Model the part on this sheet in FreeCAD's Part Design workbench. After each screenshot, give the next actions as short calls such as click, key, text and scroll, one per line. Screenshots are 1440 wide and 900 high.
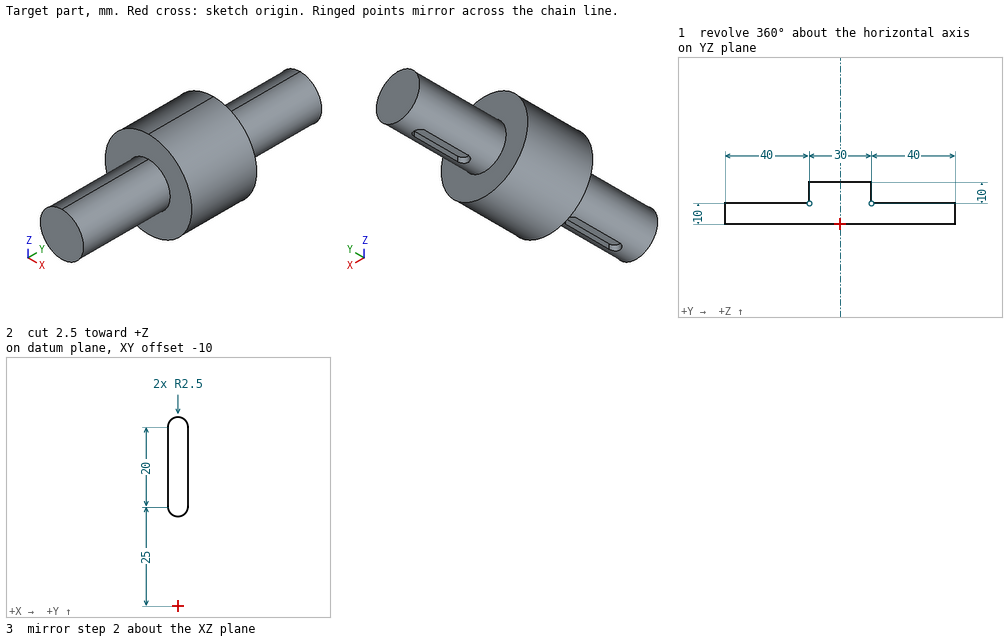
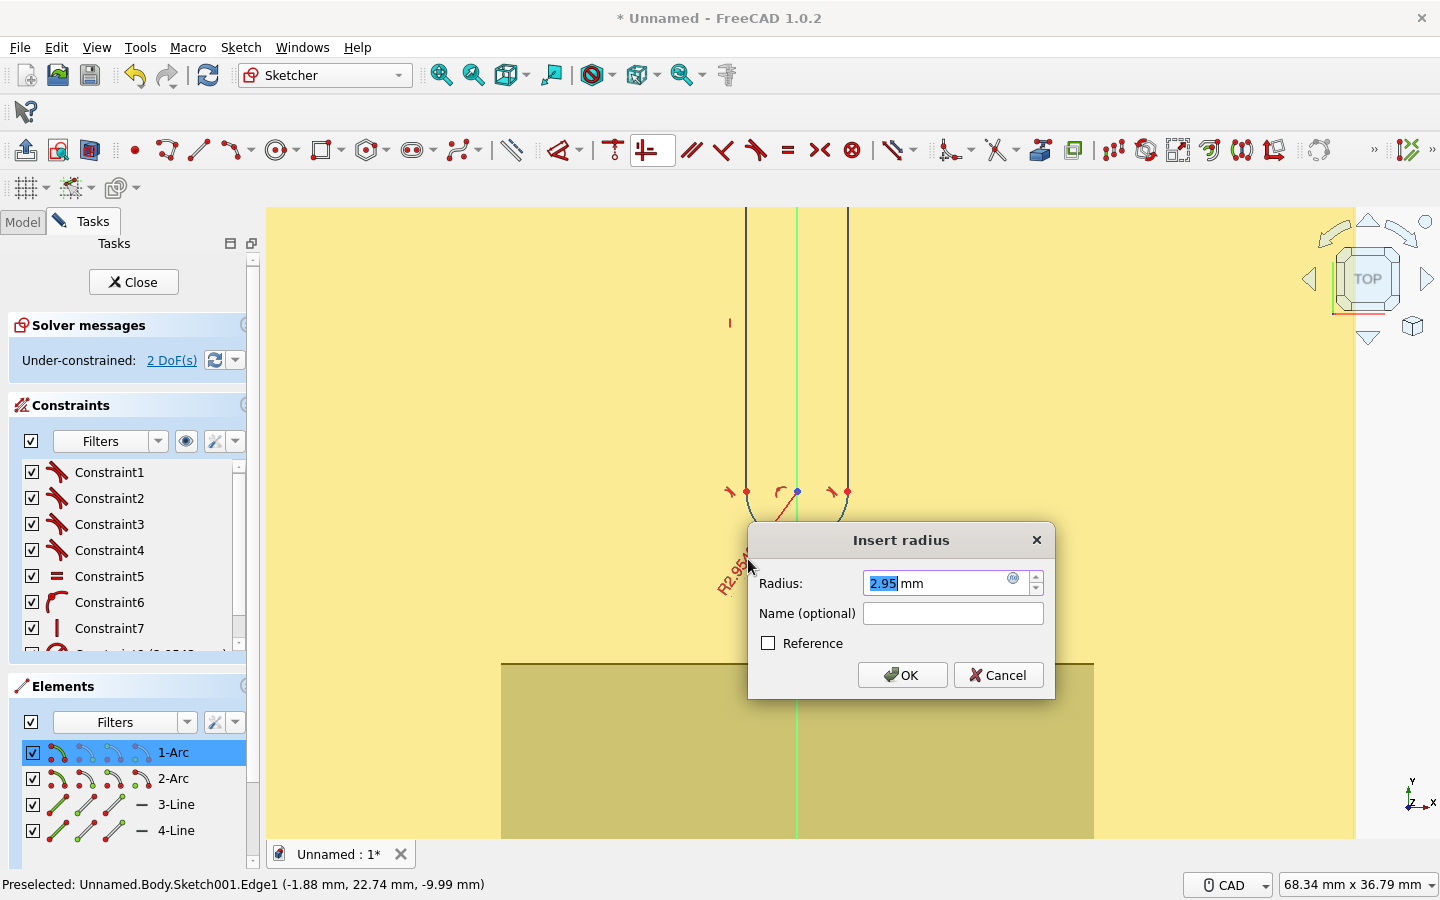
text(2.5)
key(Return)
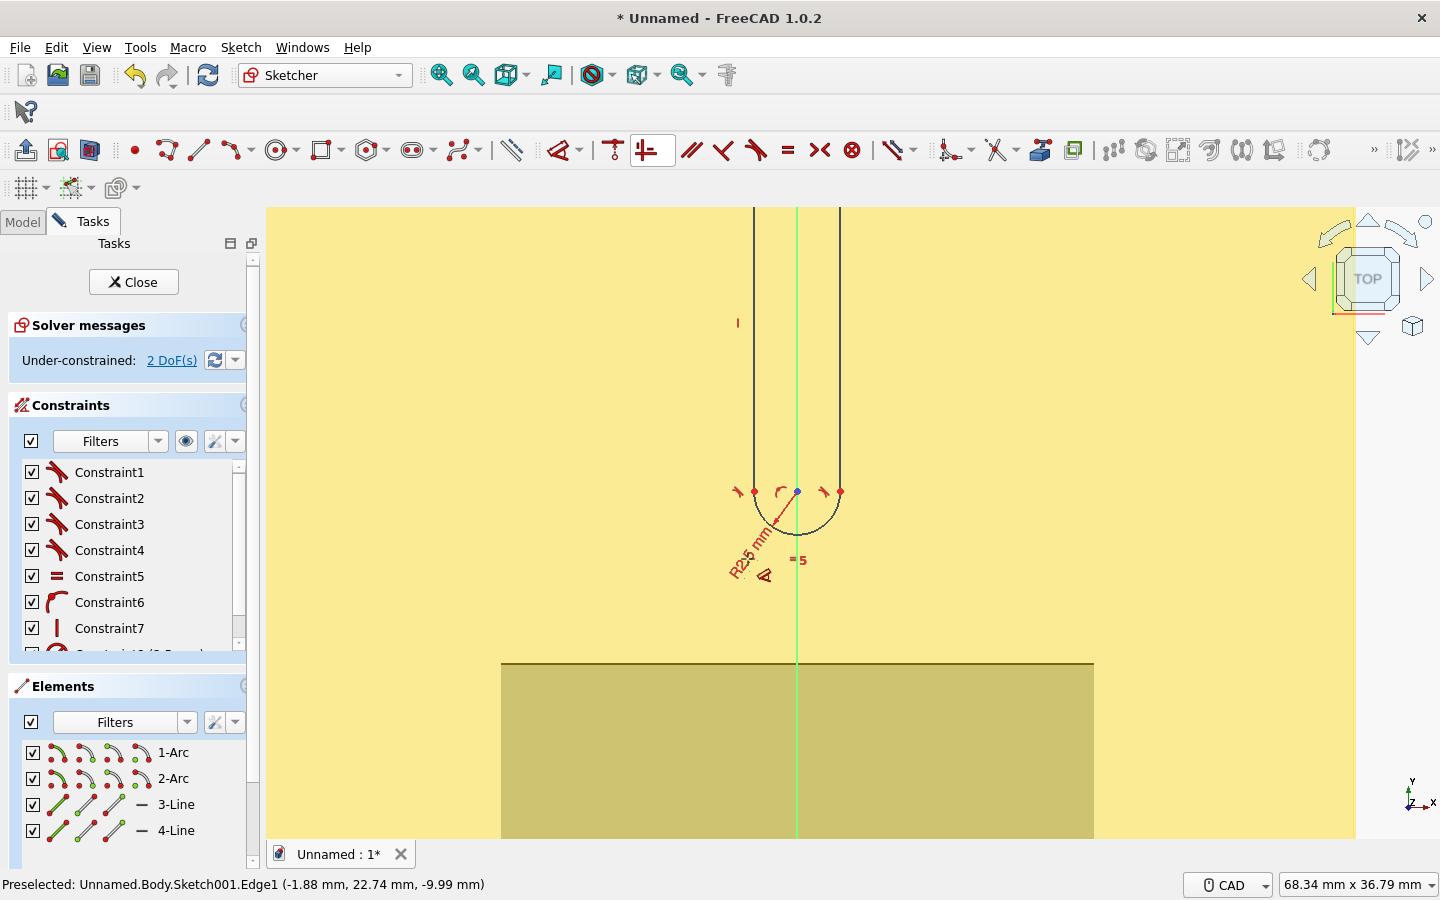
click(754, 390)
click(720, 363)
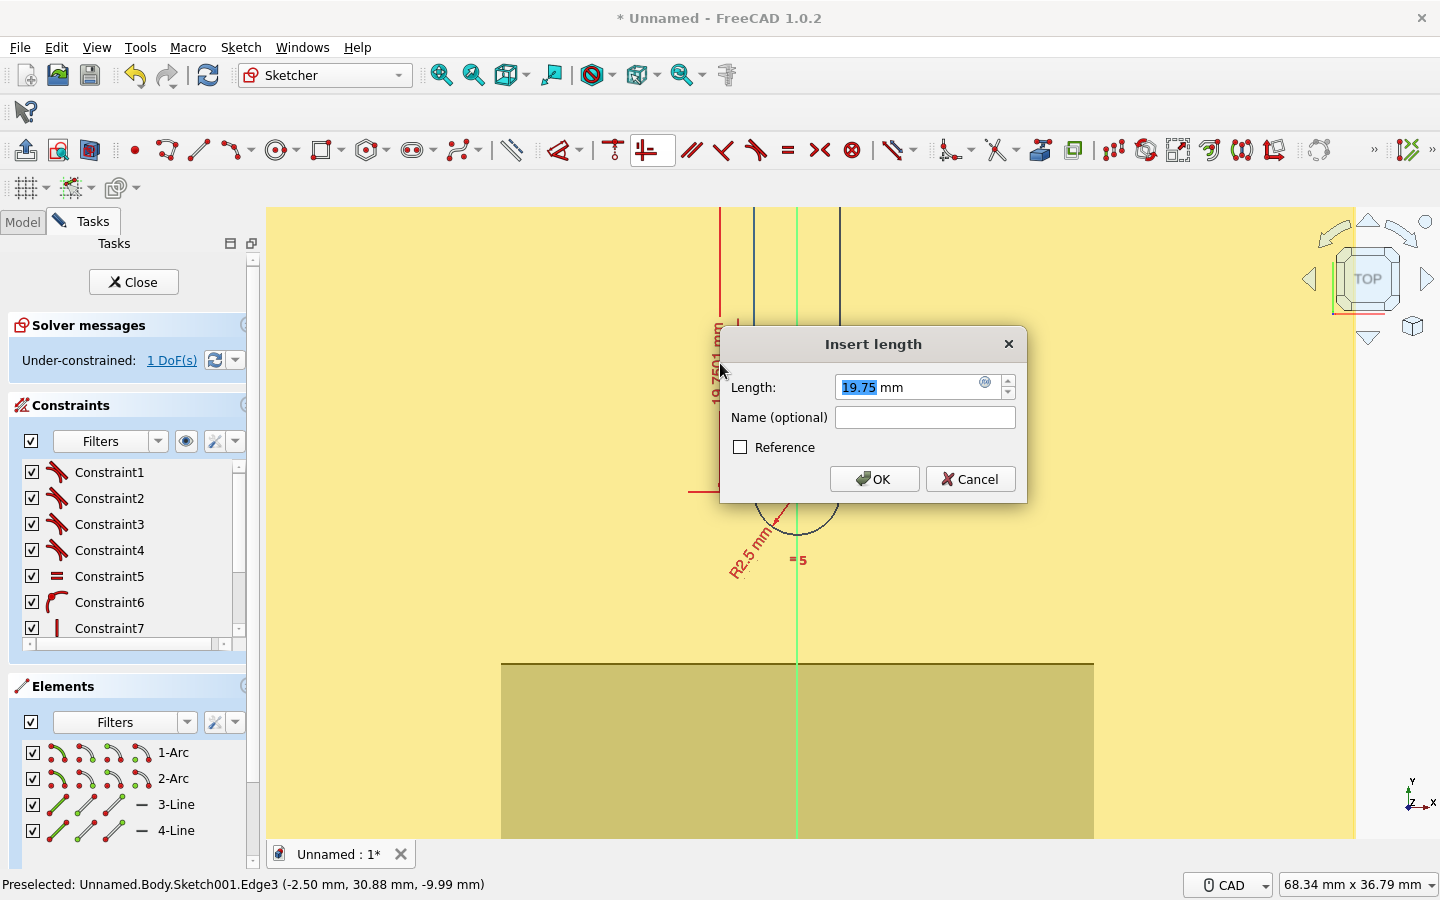
text(20)
key(Return)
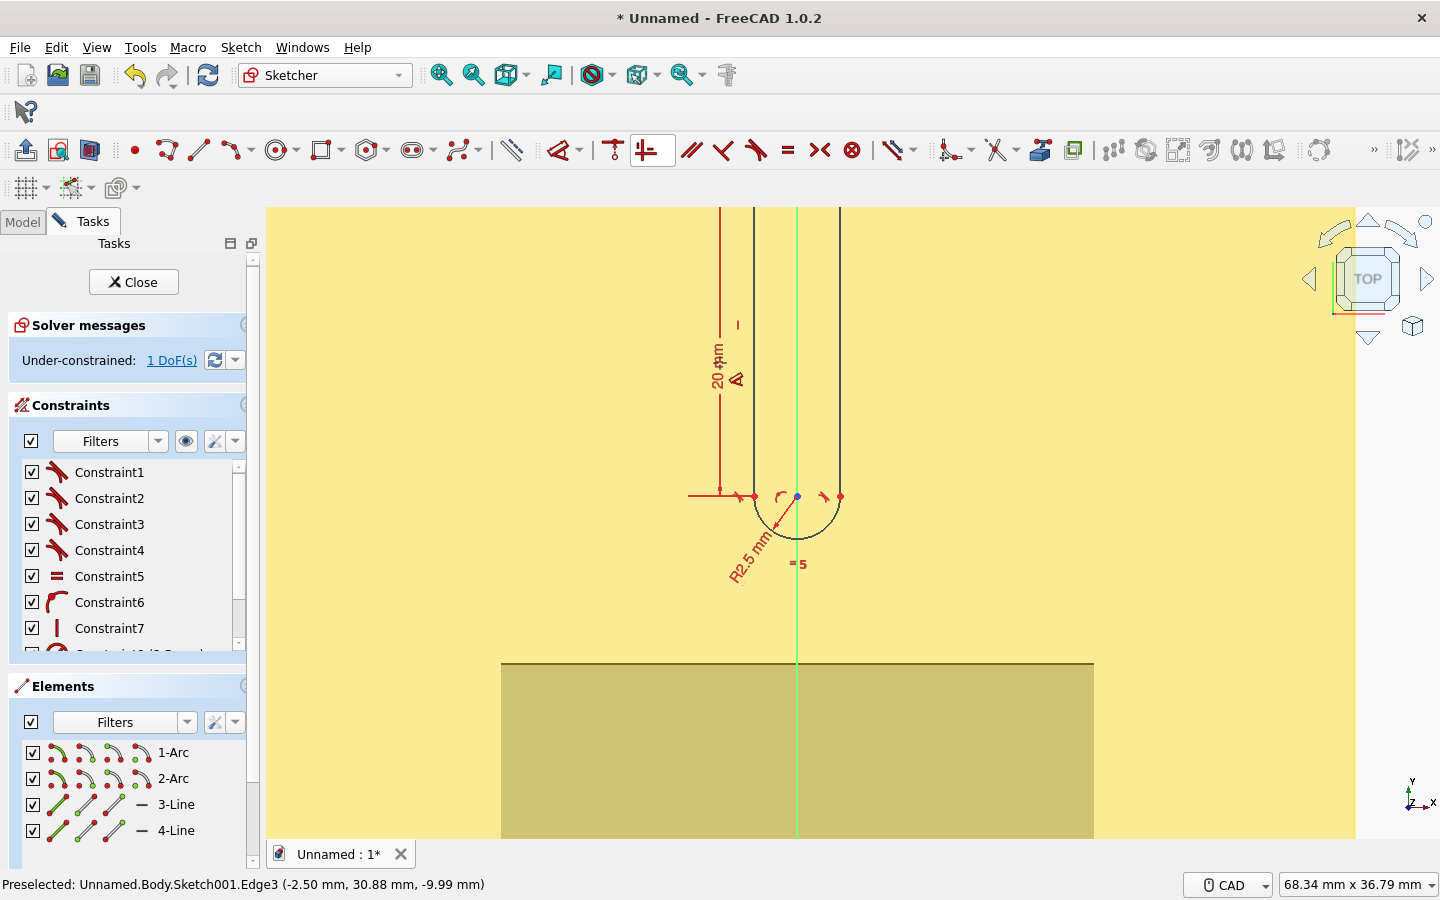
click(754, 496)
click(720, 654)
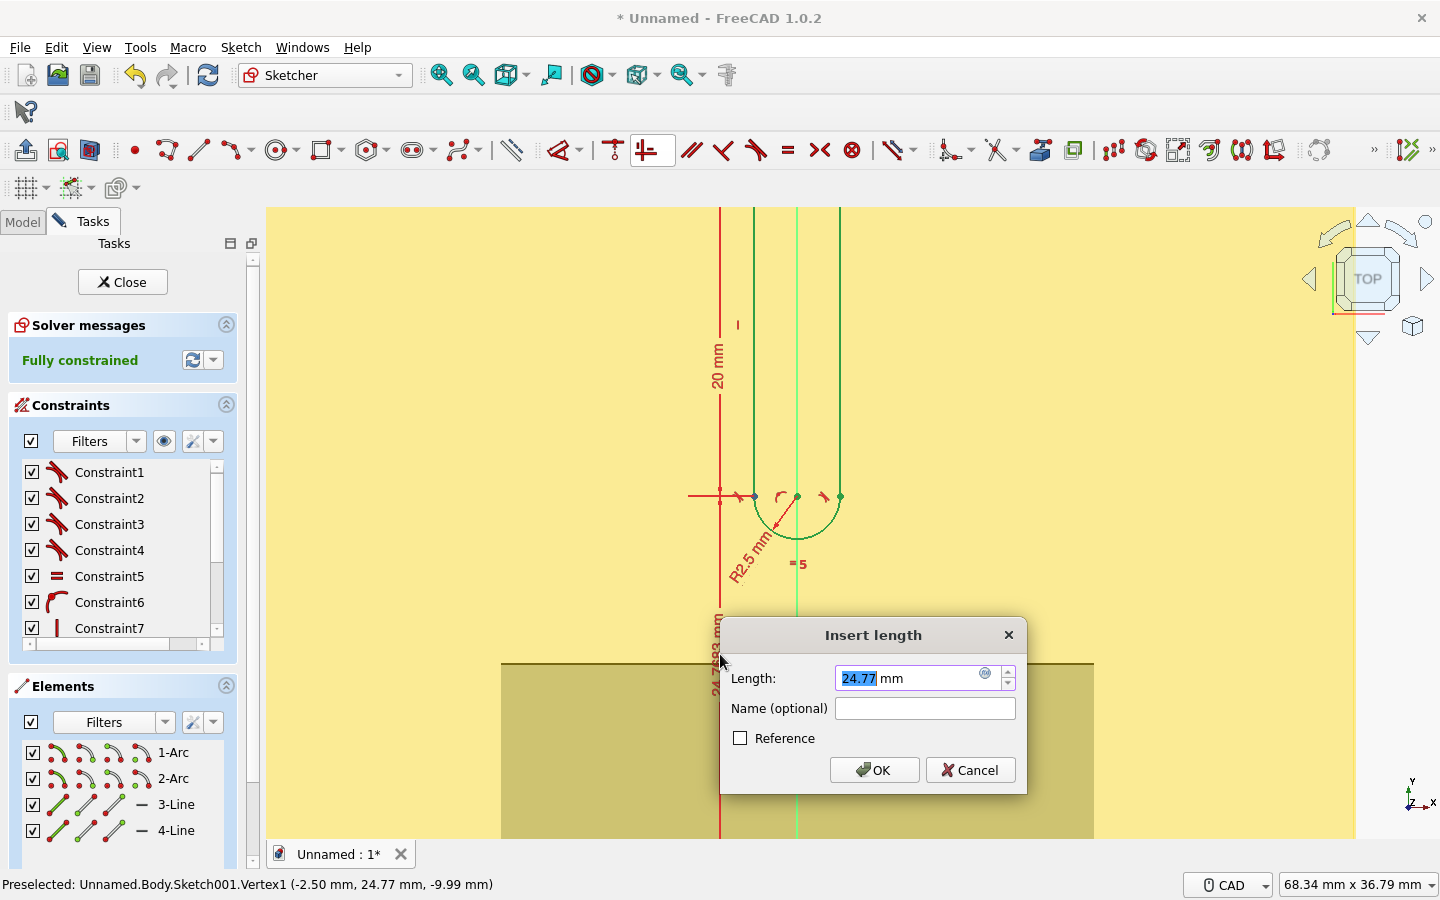
text(25)
key(Return)
key(Escape)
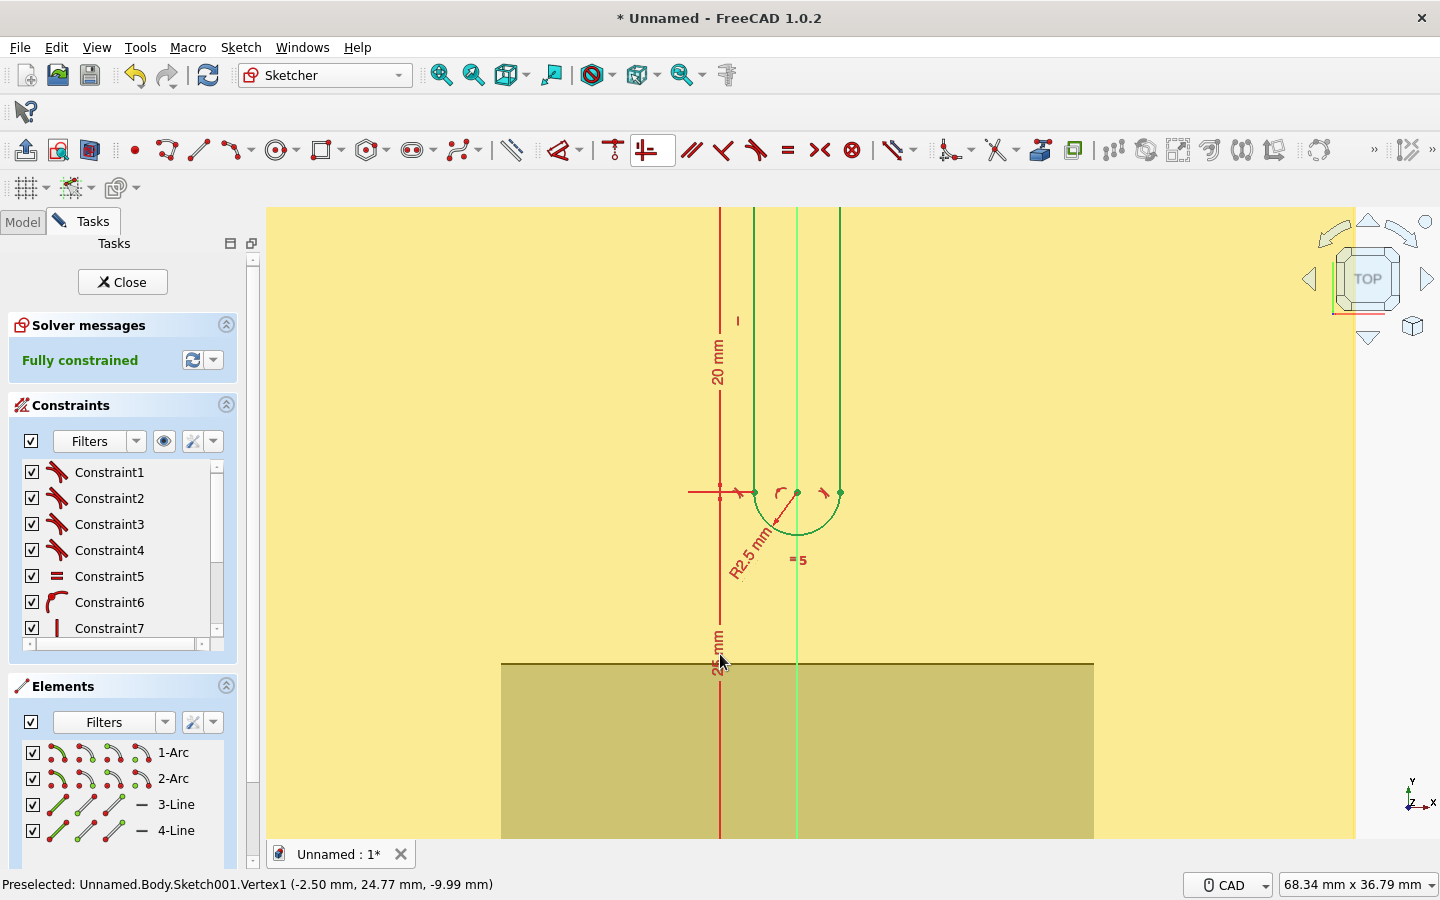
click(123, 282)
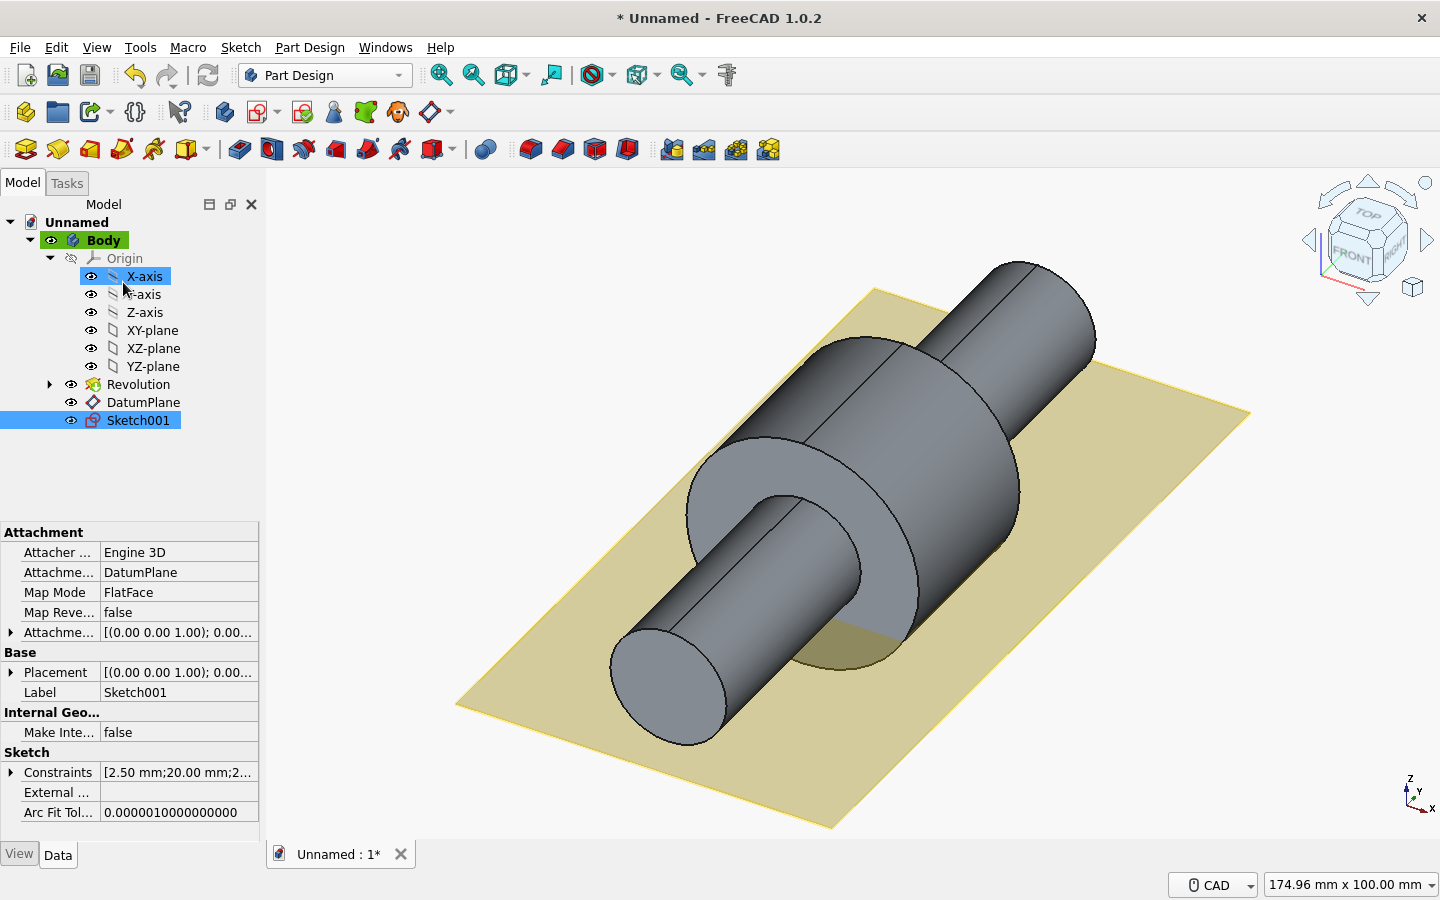
click(240, 150)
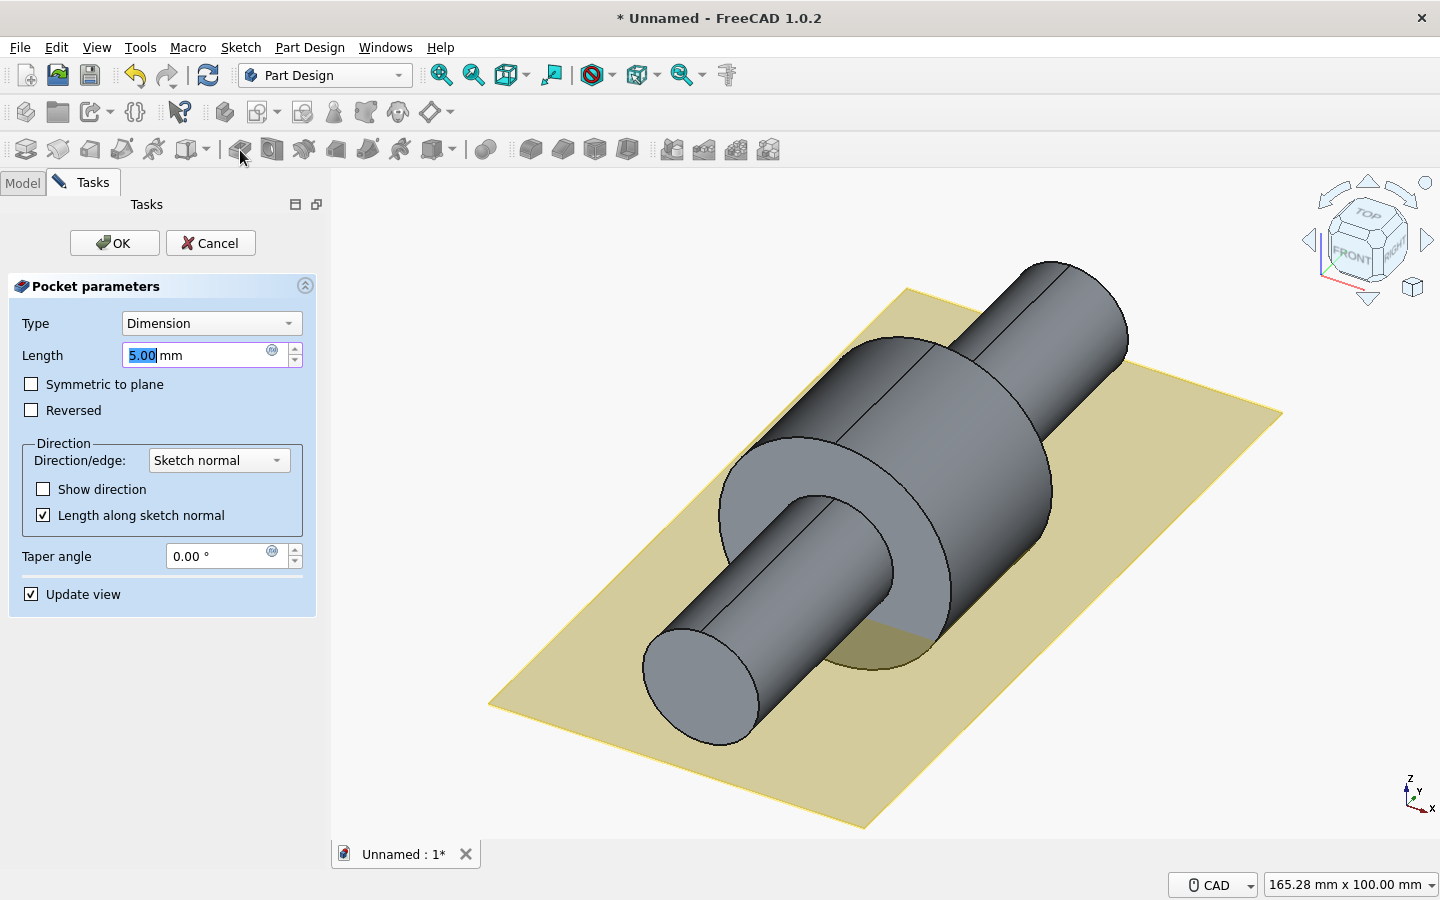
text(2.5)
key(Tab)